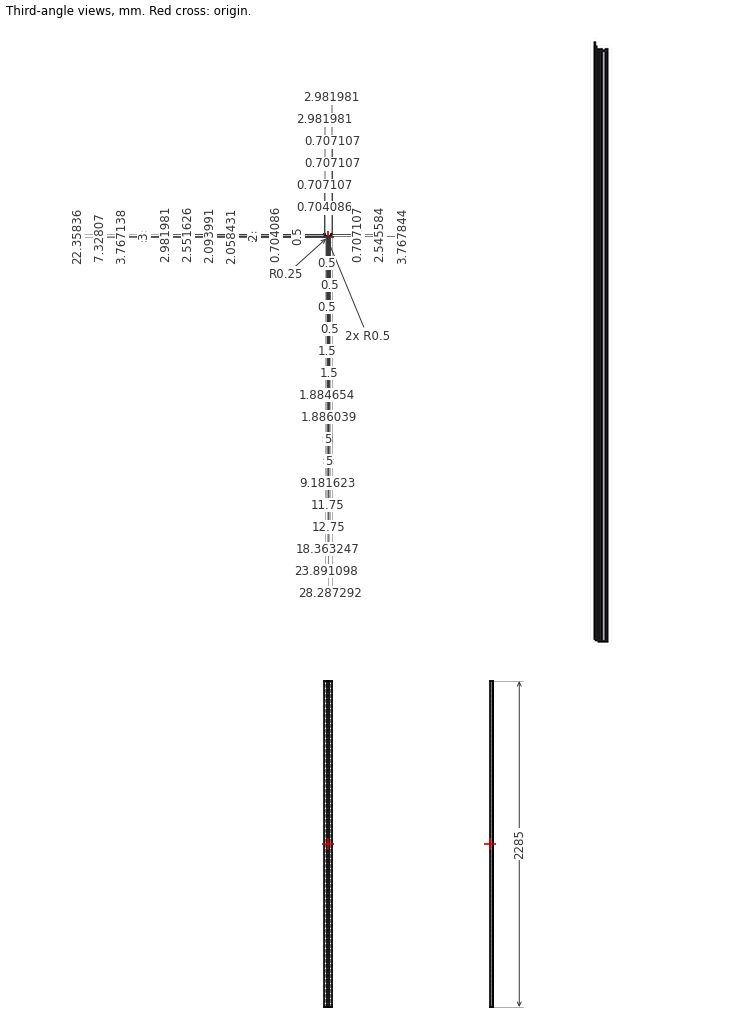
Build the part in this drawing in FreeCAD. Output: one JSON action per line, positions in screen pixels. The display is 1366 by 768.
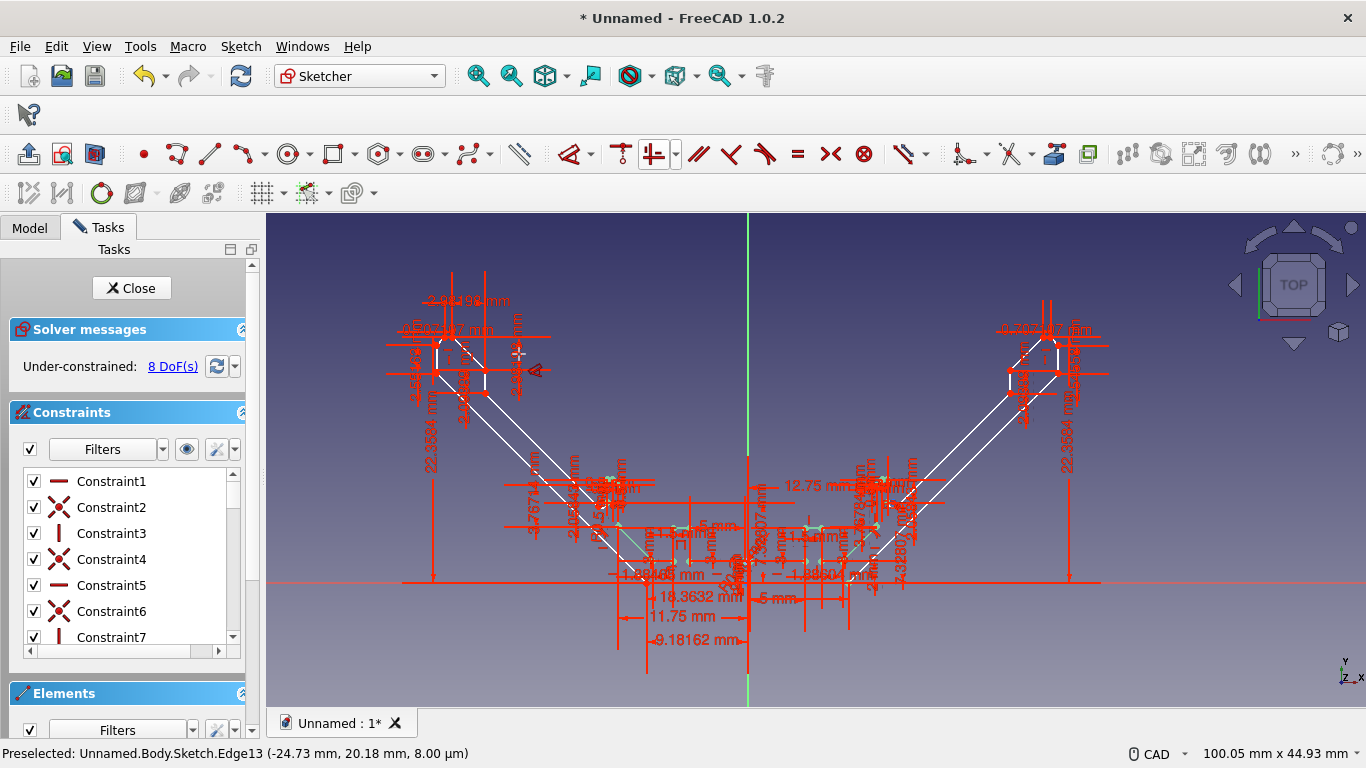
{"action": "scroll", "coordinate": [441, 341], "scroll_direction": "up", "scroll_amount": 9}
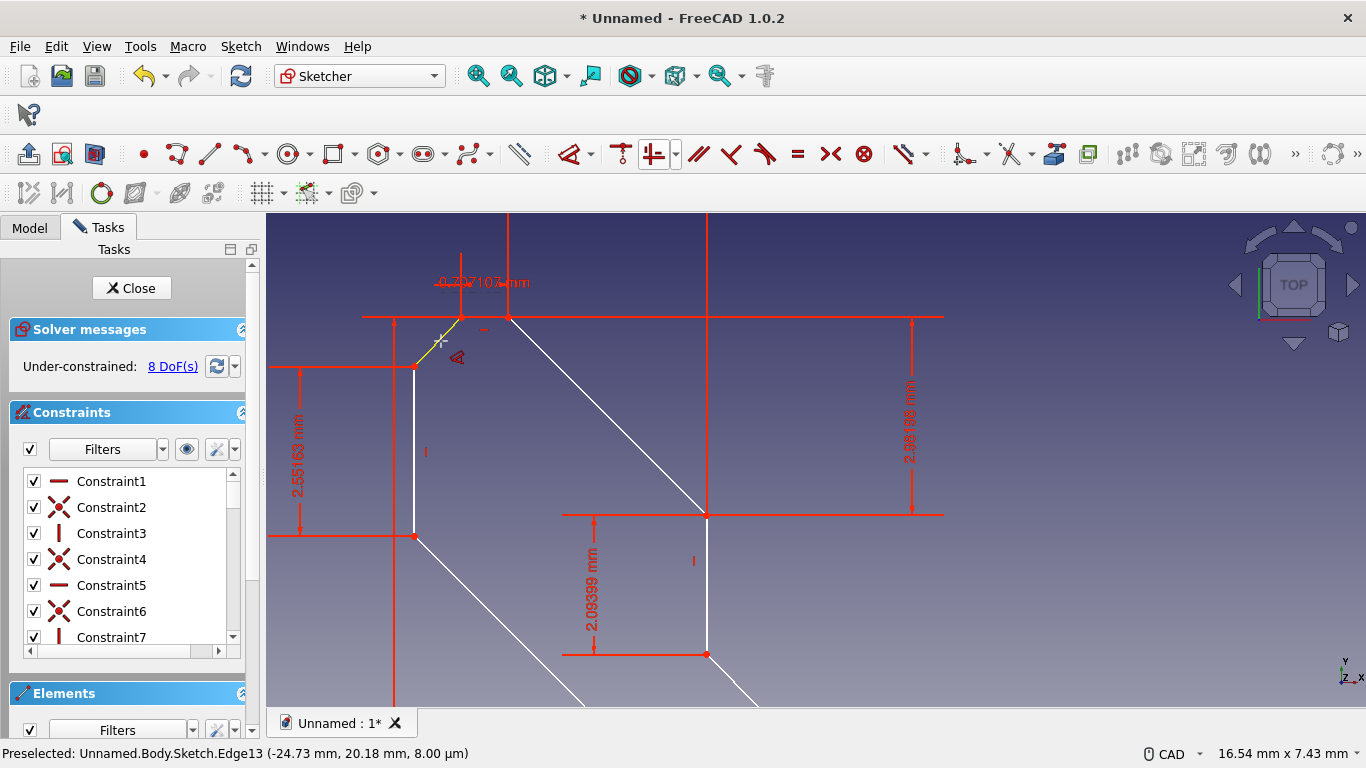
{"action": "left_click", "coordinate": [438, 342]}
{"action": "left_click", "coordinate": [438, 401]}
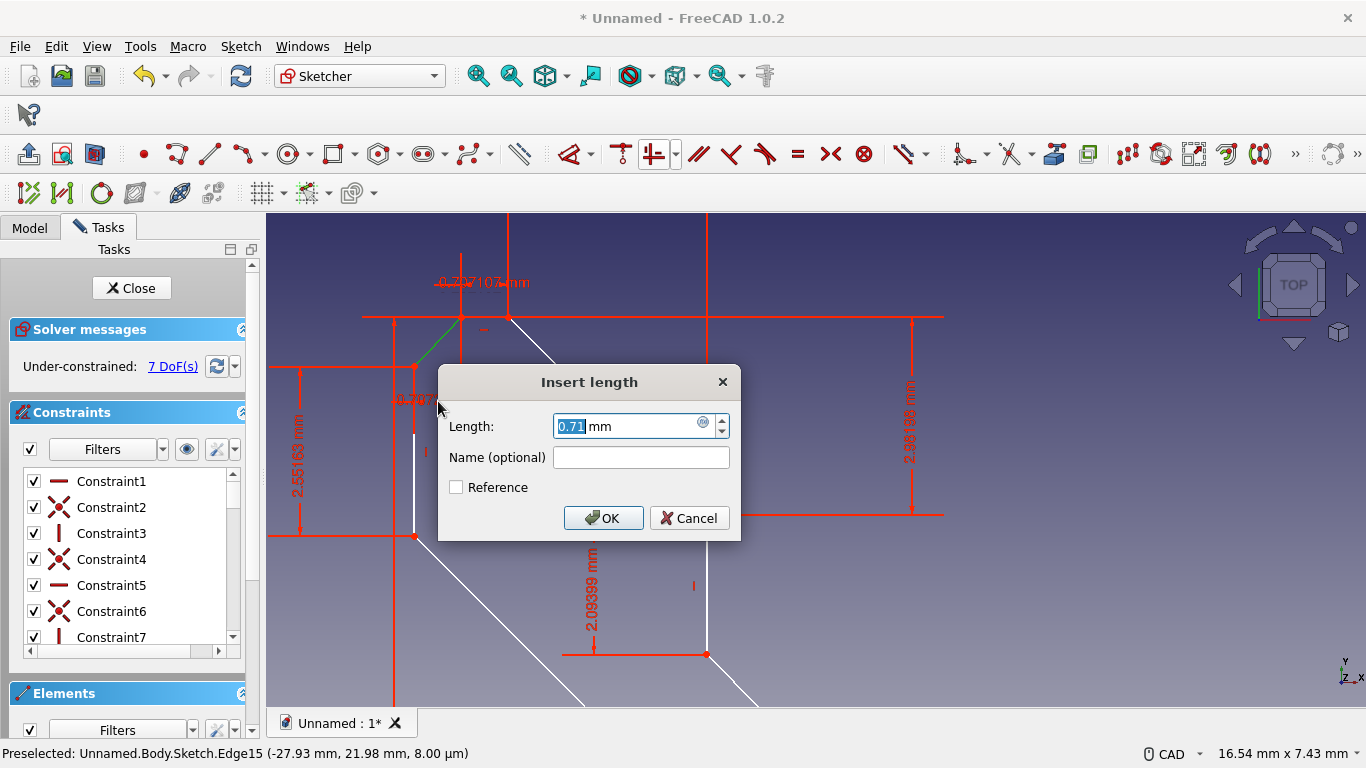
{"action": "type", "text": "0.704086"}
{"action": "key", "text": "Return"}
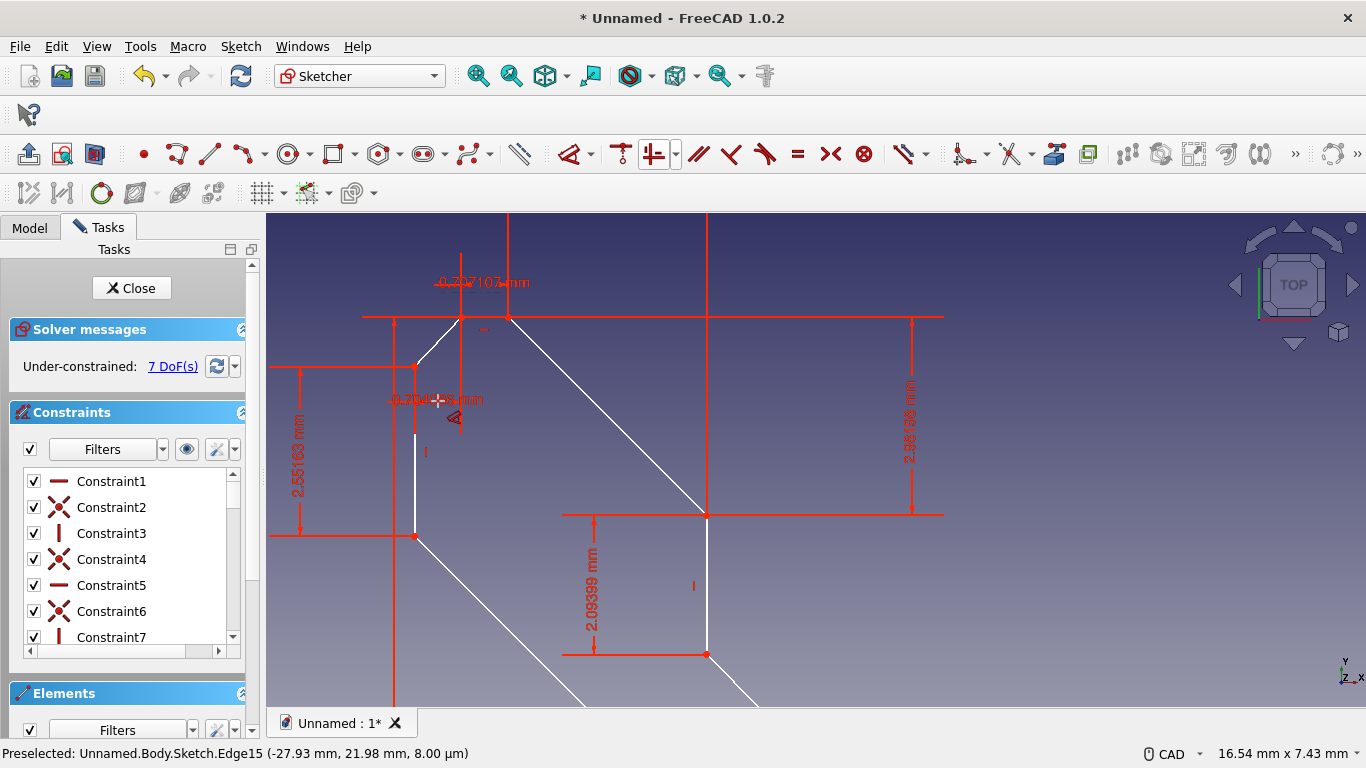
{"action": "left_click", "coordinate": [447, 332]}
{"action": "left_click", "coordinate": [381, 342]}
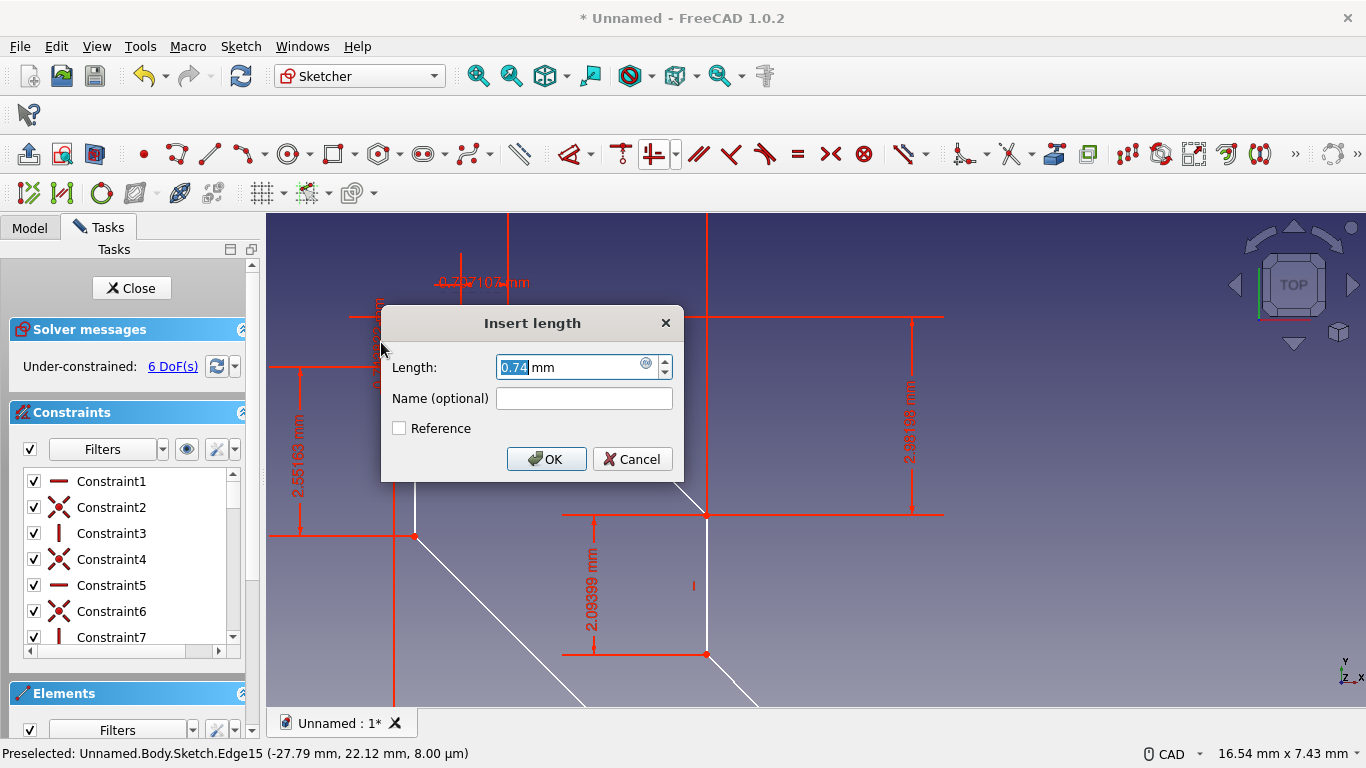
{"action": "type", "text": "0.704086"}
{"action": "key", "text": "Return"}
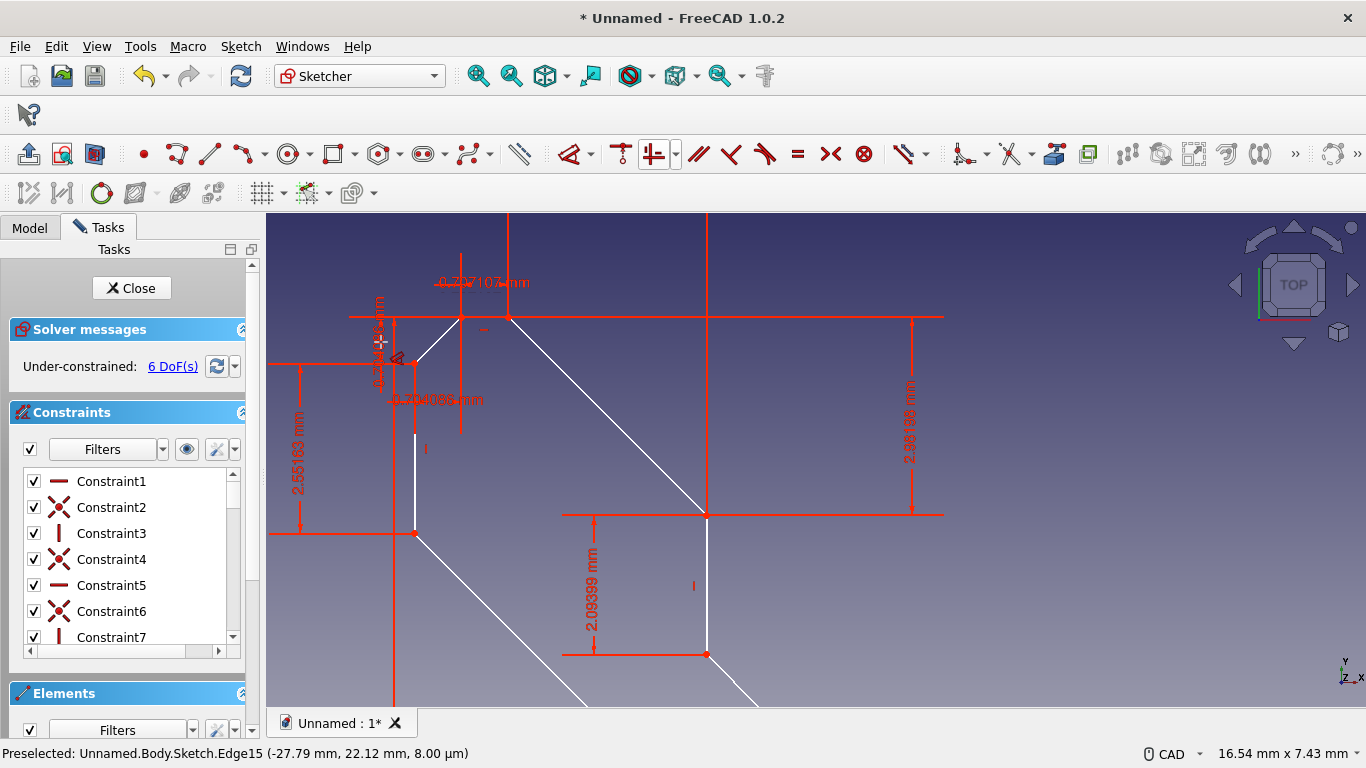
{"action": "scroll", "coordinate": [441, 341], "scroll_direction": "down", "scroll_amount": 9}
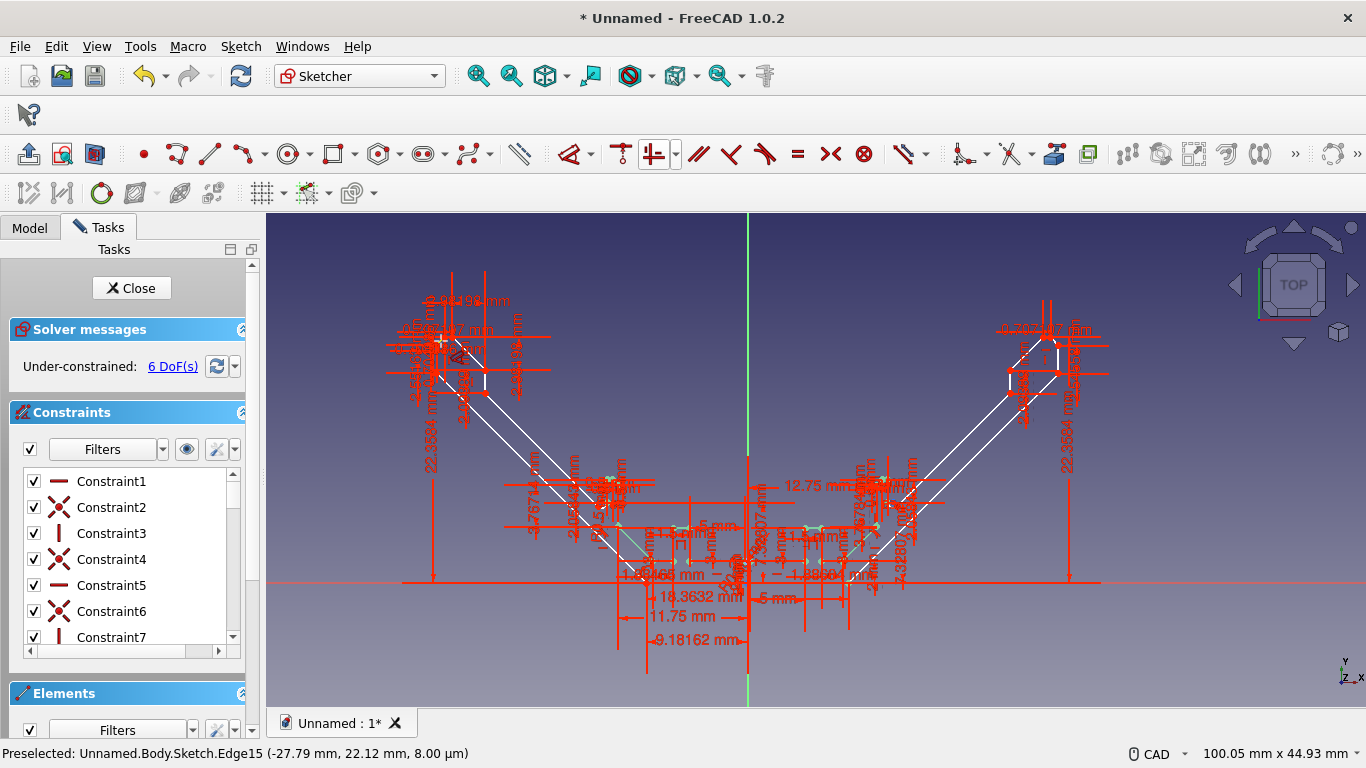
{"action": "scroll", "coordinate": [1056, 343], "scroll_direction": "up", "scroll_amount": 9}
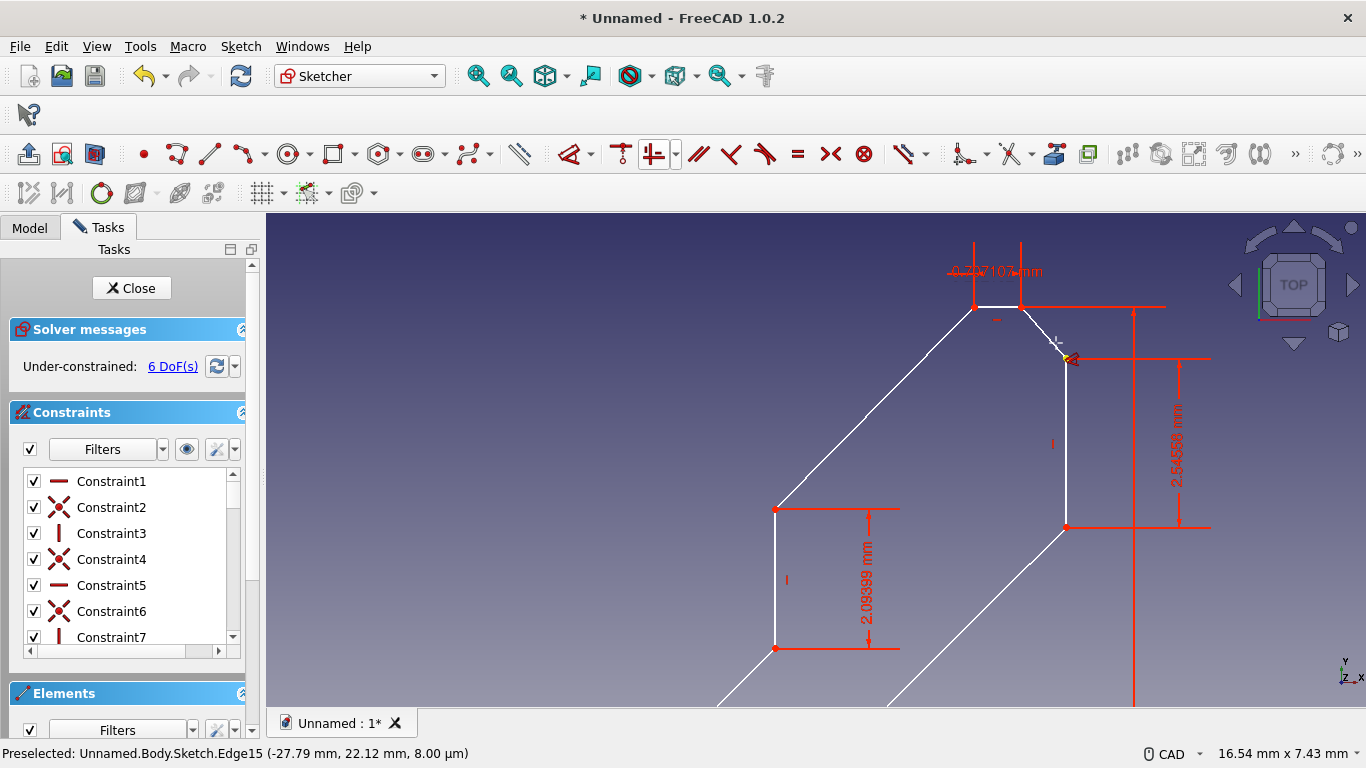
{"action": "left_click", "coordinate": [1053, 343]}
{"action": "left_click", "coordinate": [1044, 393]}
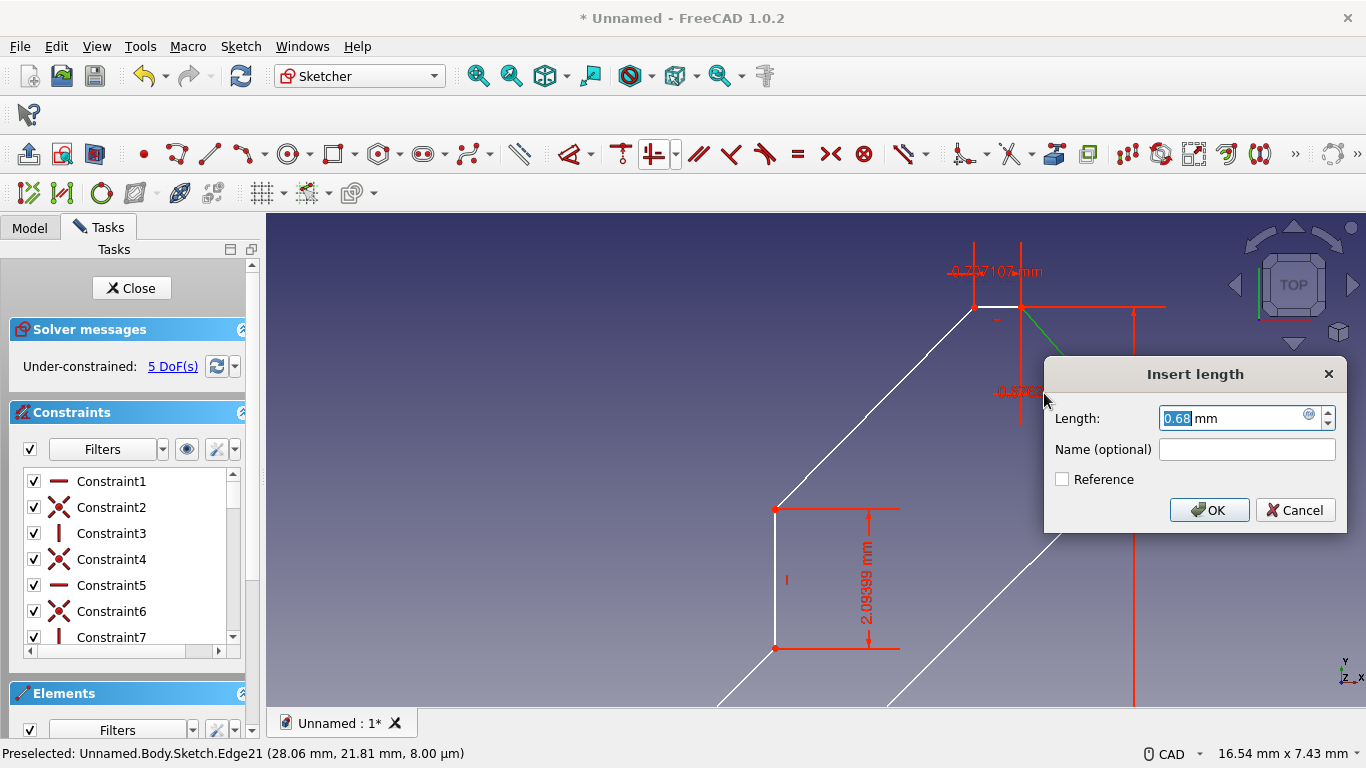
{"action": "type", "text": "0.707107"}
{"action": "key", "text": "Return"}